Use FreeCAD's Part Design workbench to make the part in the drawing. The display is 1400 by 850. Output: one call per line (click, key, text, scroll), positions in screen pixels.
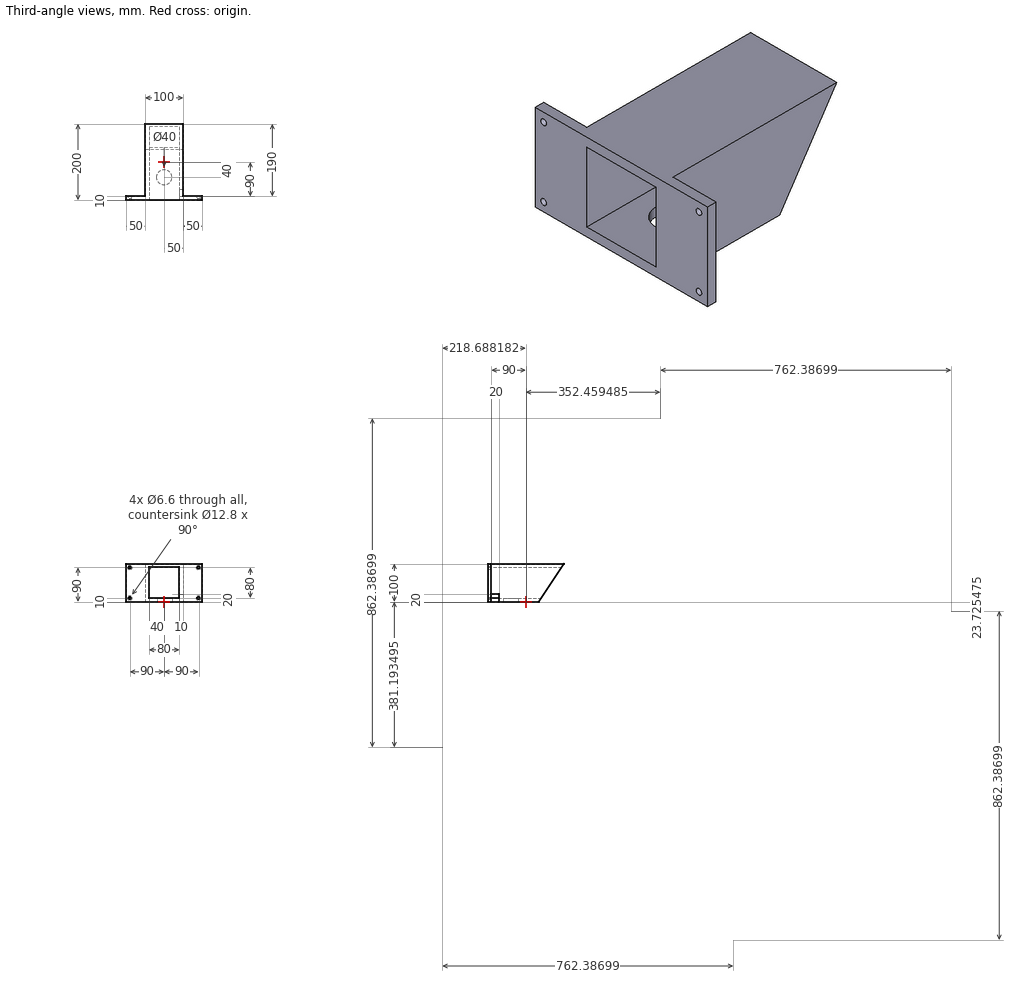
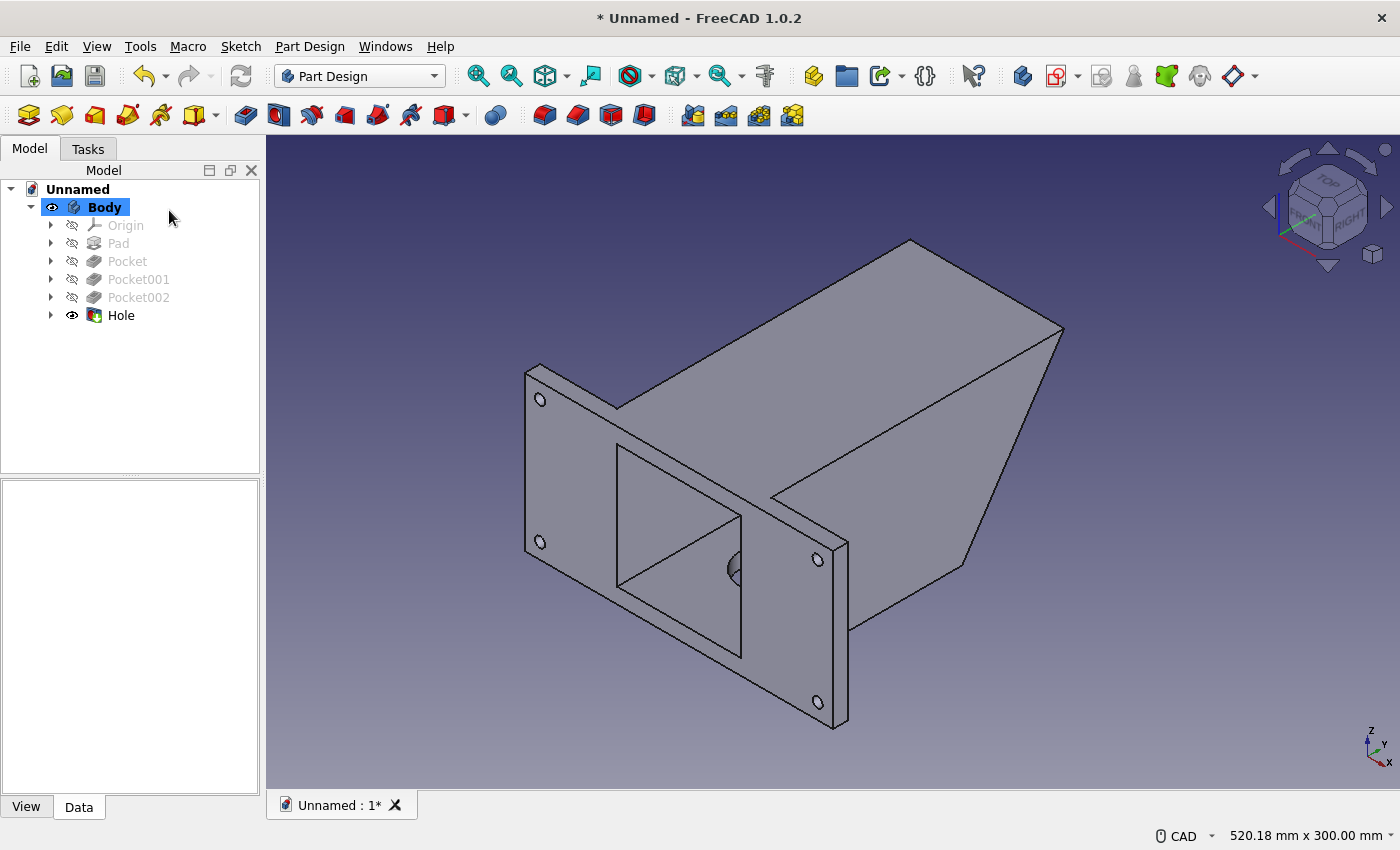
click(918, 501)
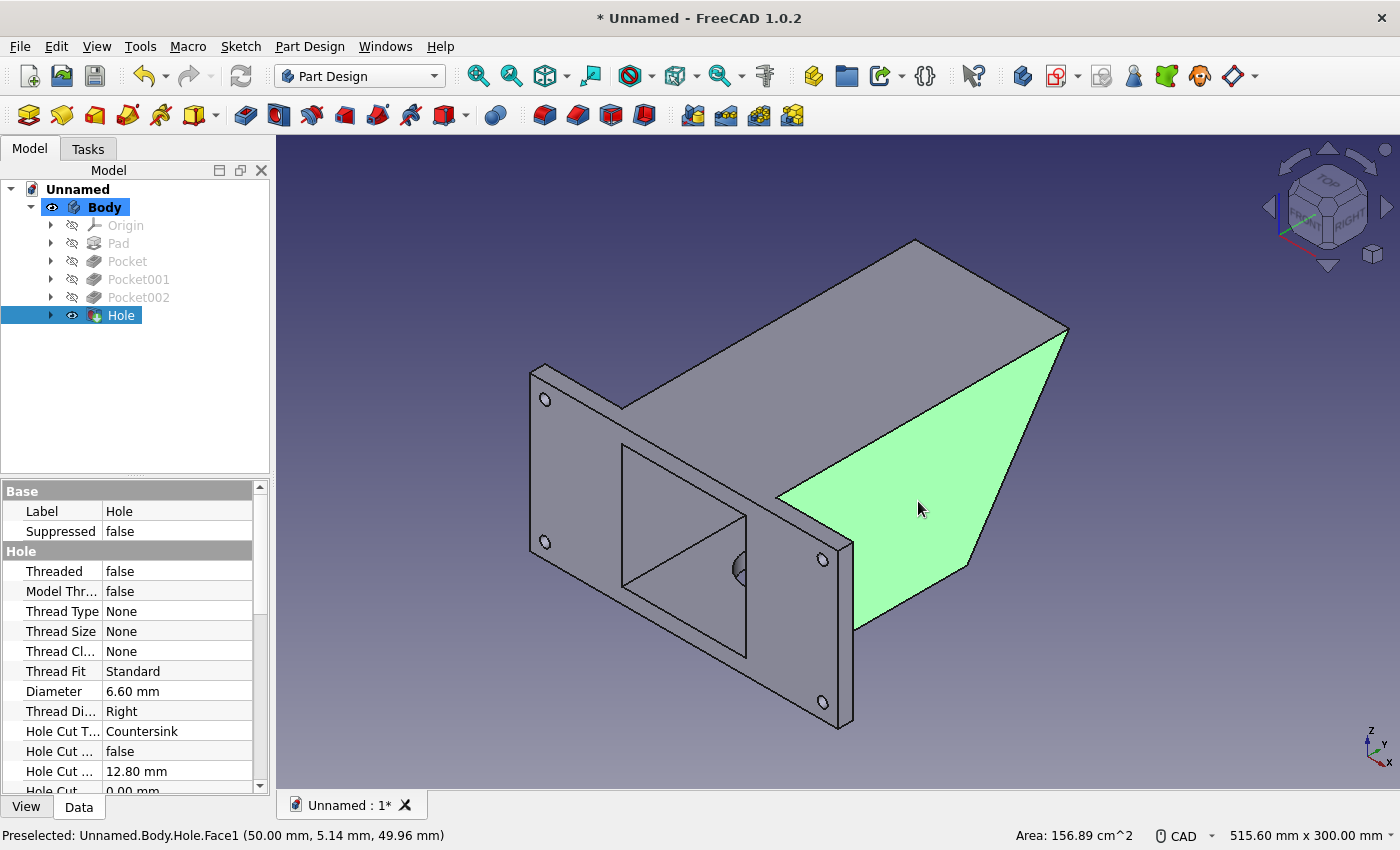
click(1056, 76)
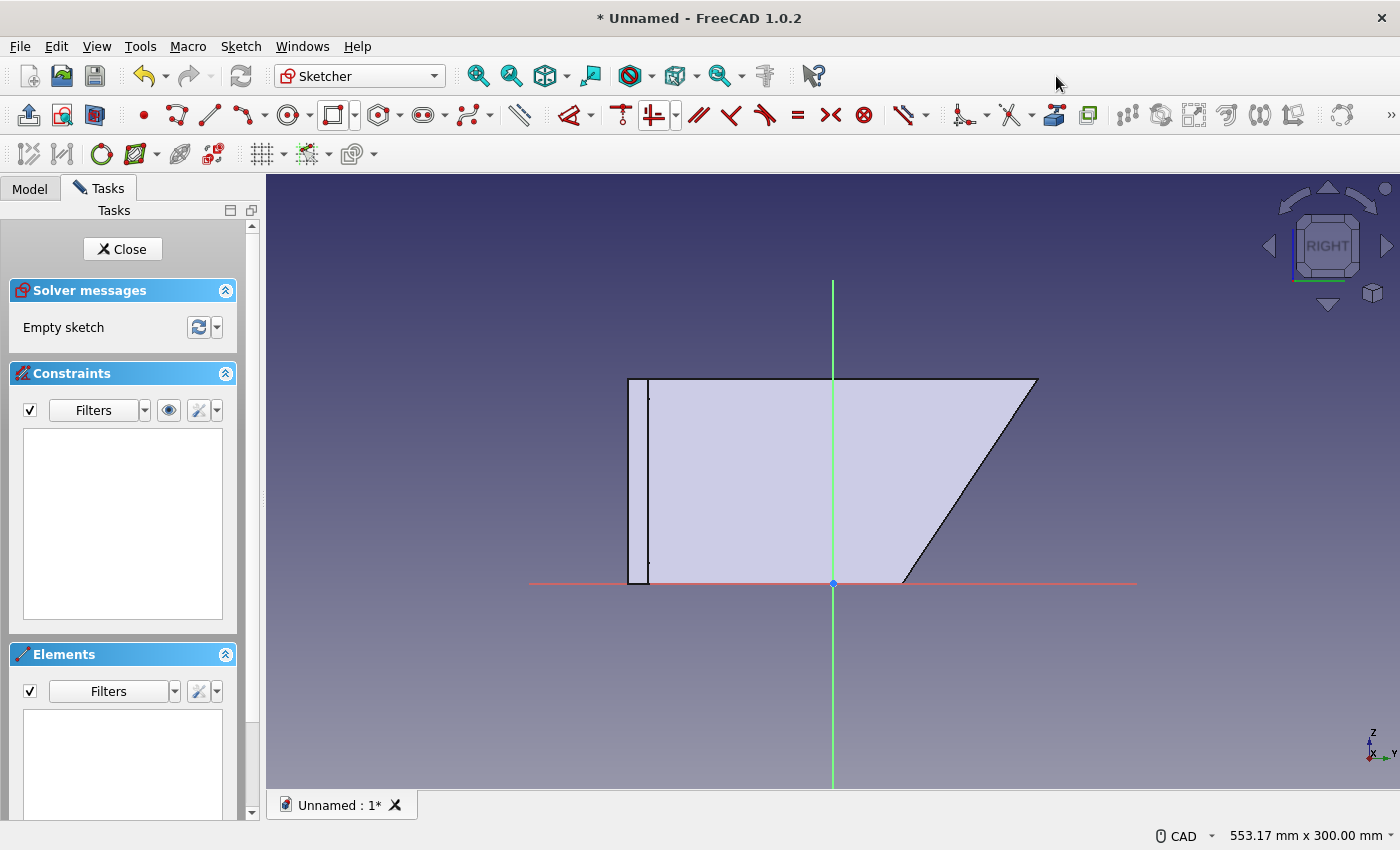
scroll(657, 574, up, 11)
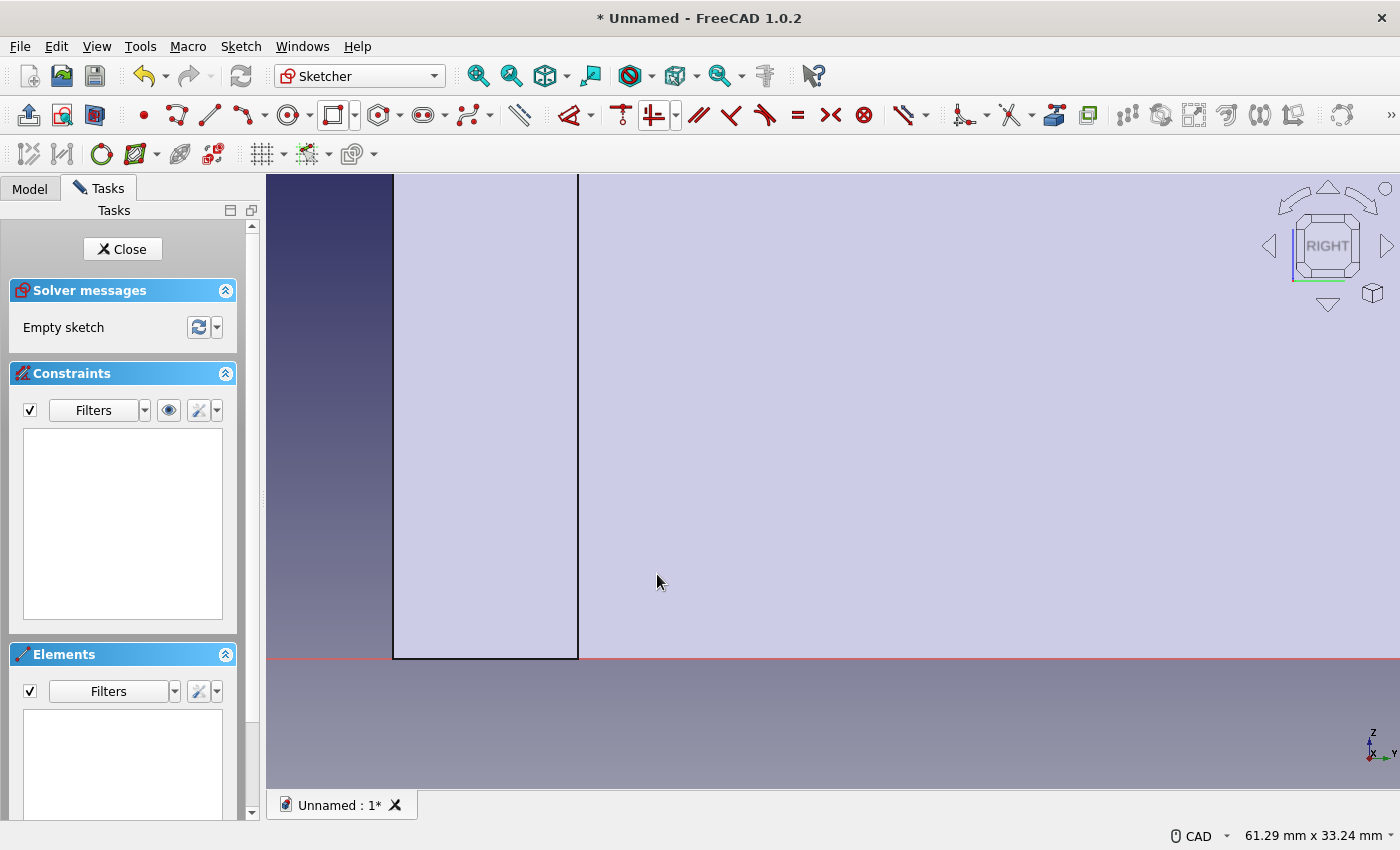
click(332, 116)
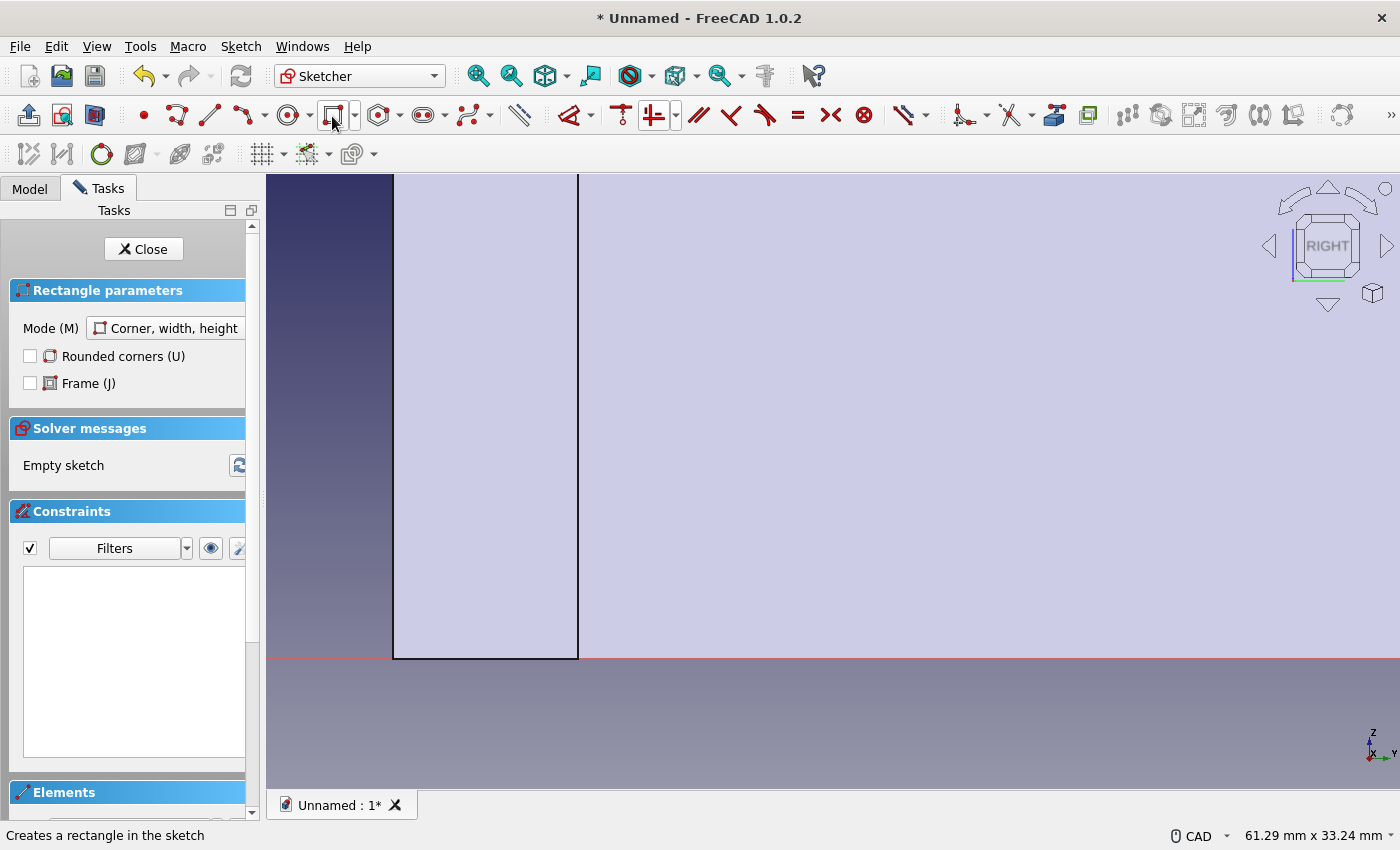
click(578, 289)
click(948, 659)
key(Escape)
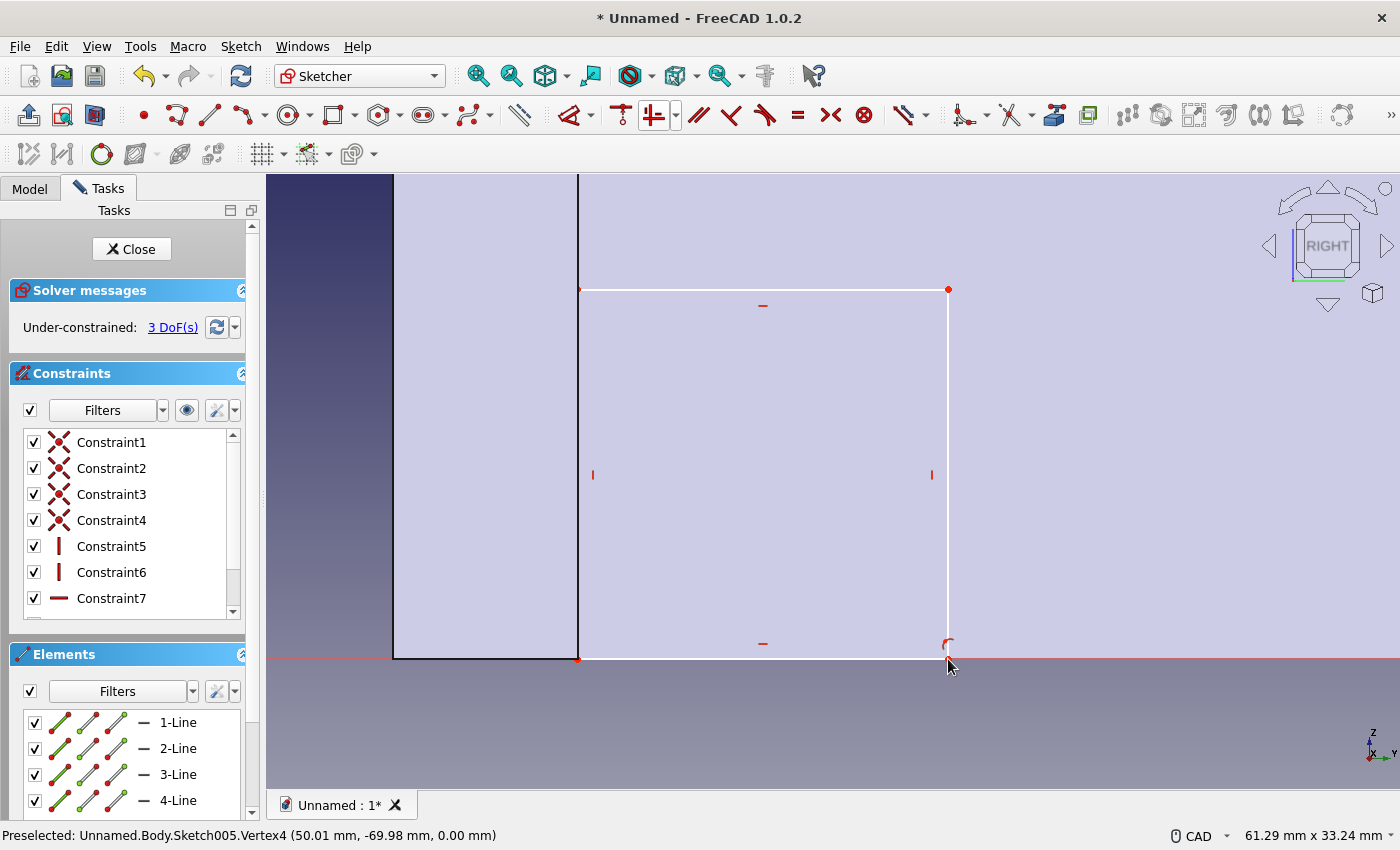
click(568, 116)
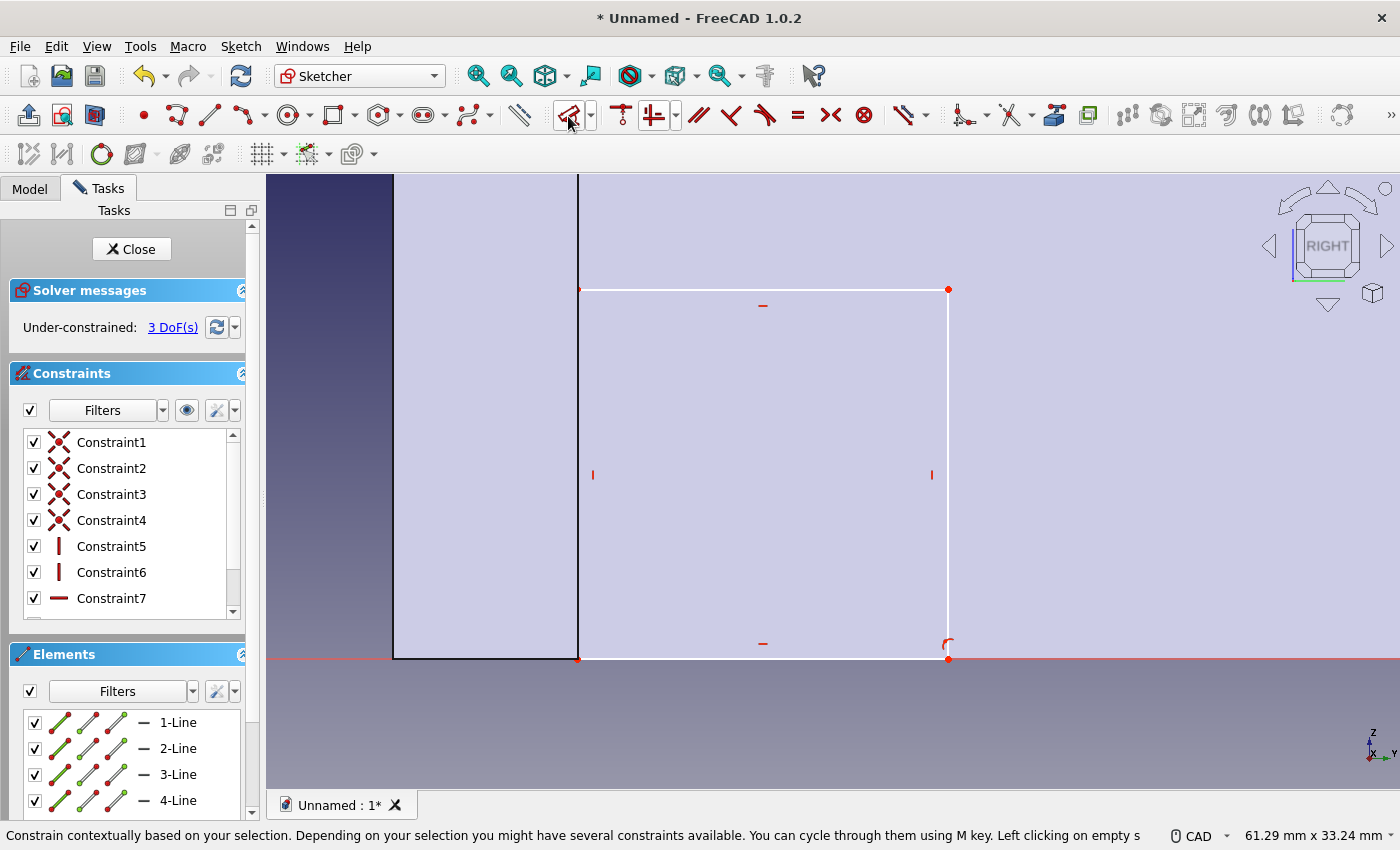
click(578, 401)
click(544, 475)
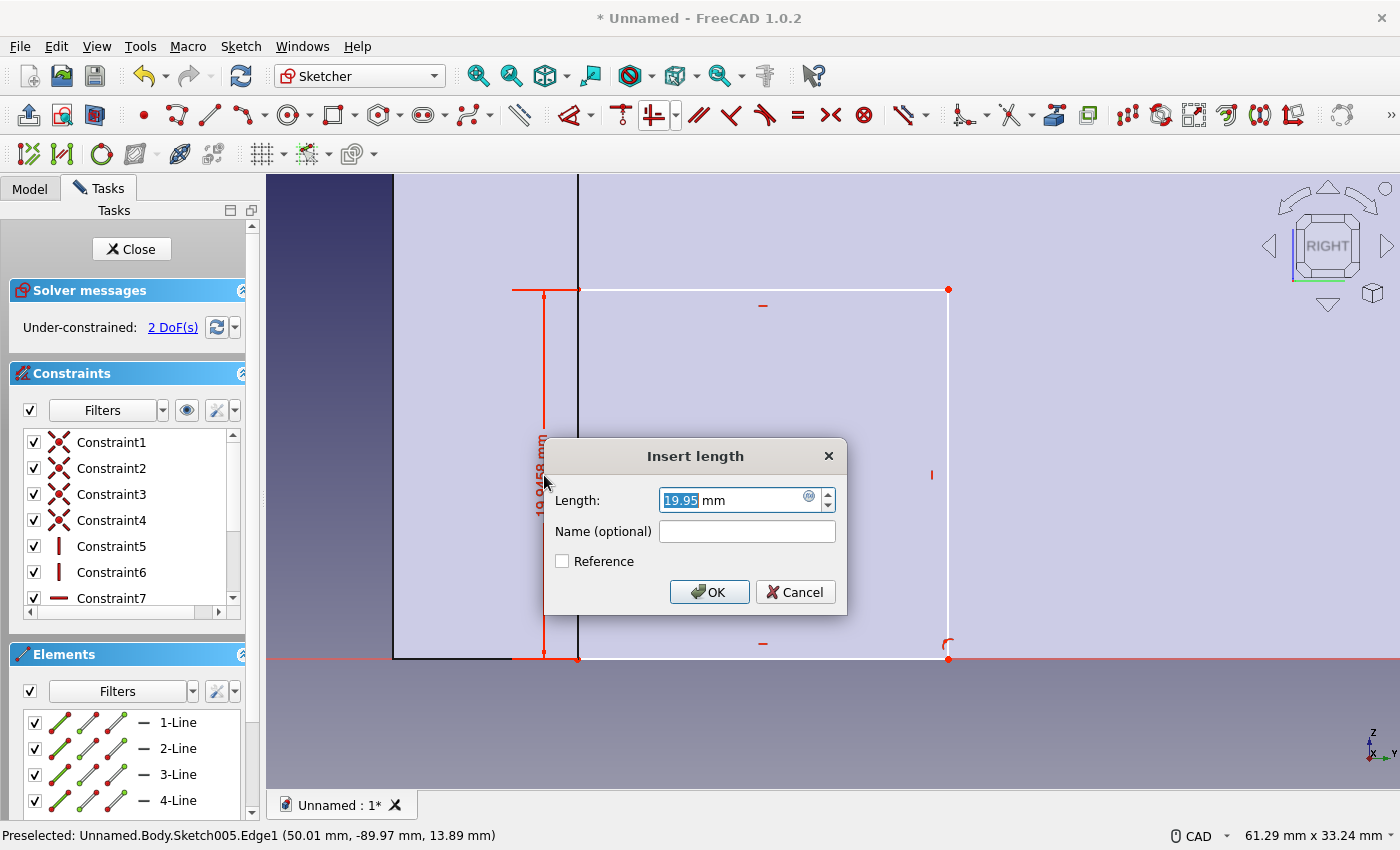
text(20)
key(Return)